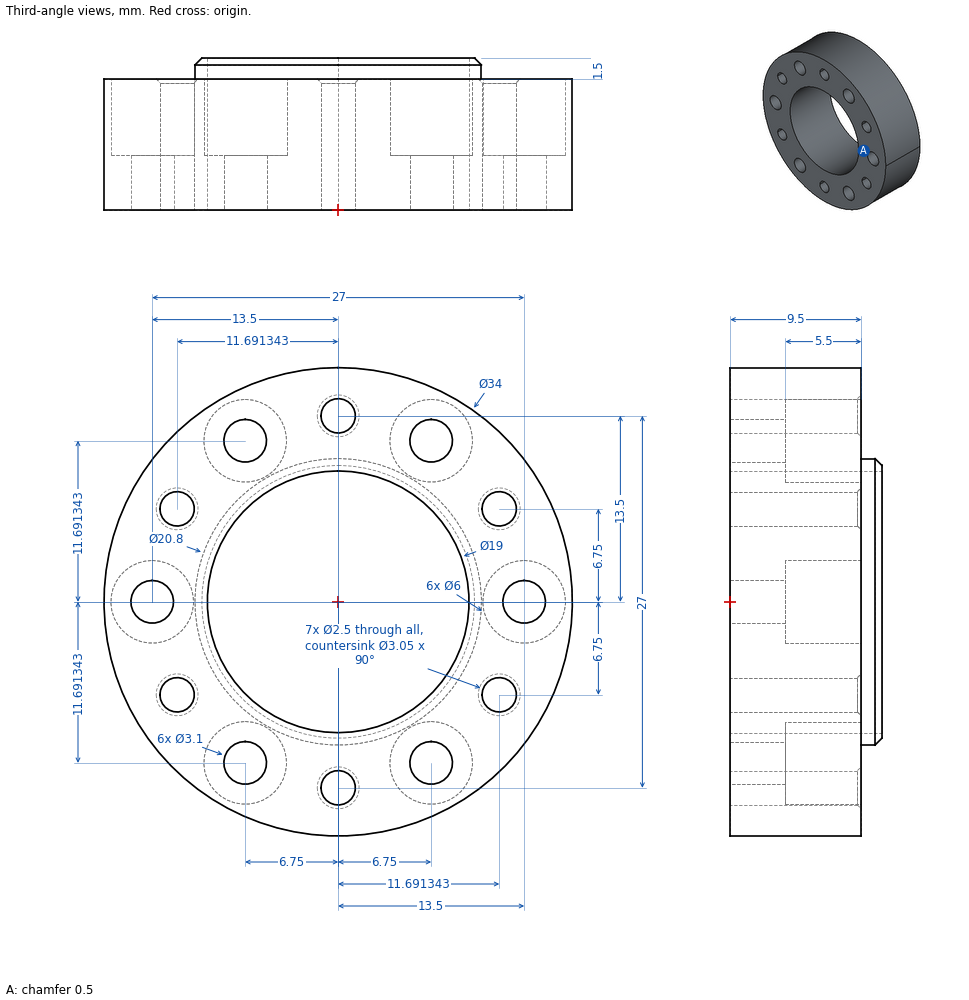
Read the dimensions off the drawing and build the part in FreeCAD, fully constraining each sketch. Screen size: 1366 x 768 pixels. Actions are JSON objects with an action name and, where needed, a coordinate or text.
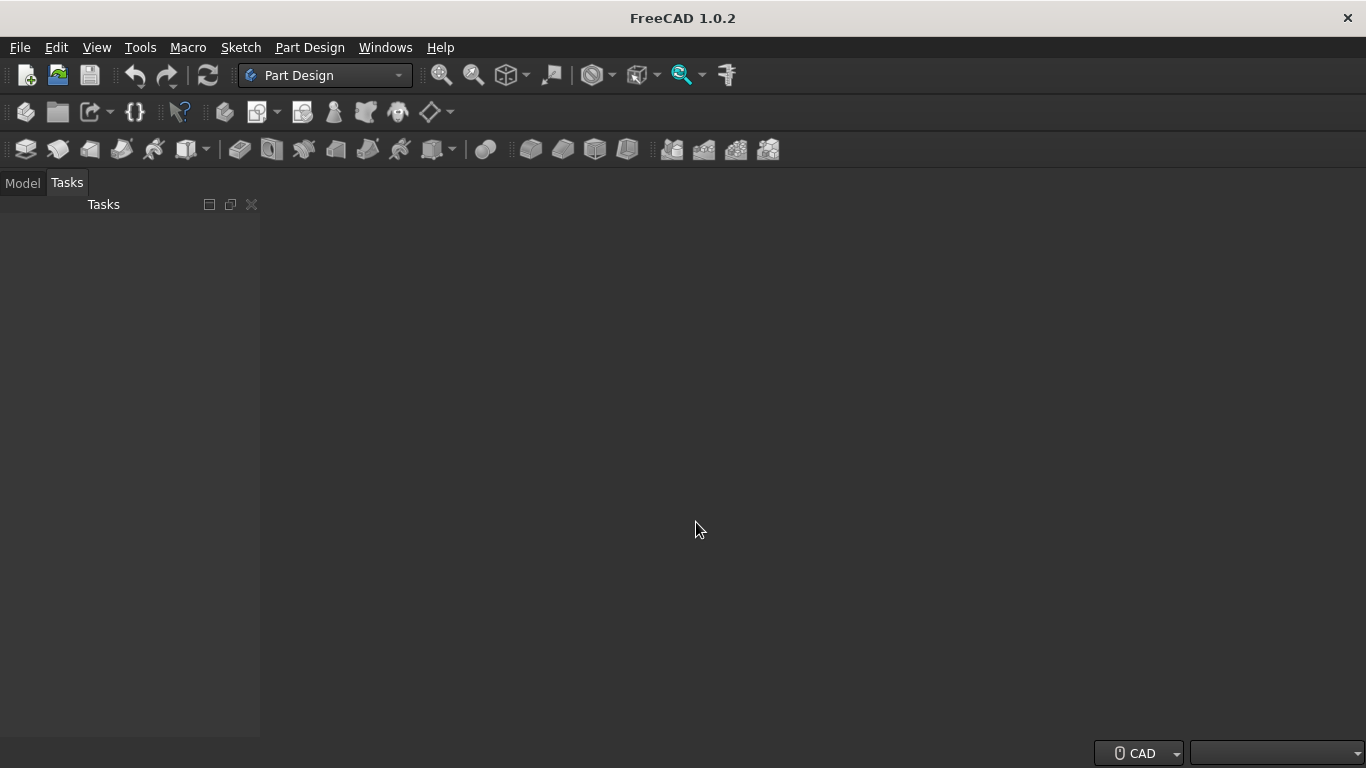
{"action": "left_click", "coordinate": [26, 76]}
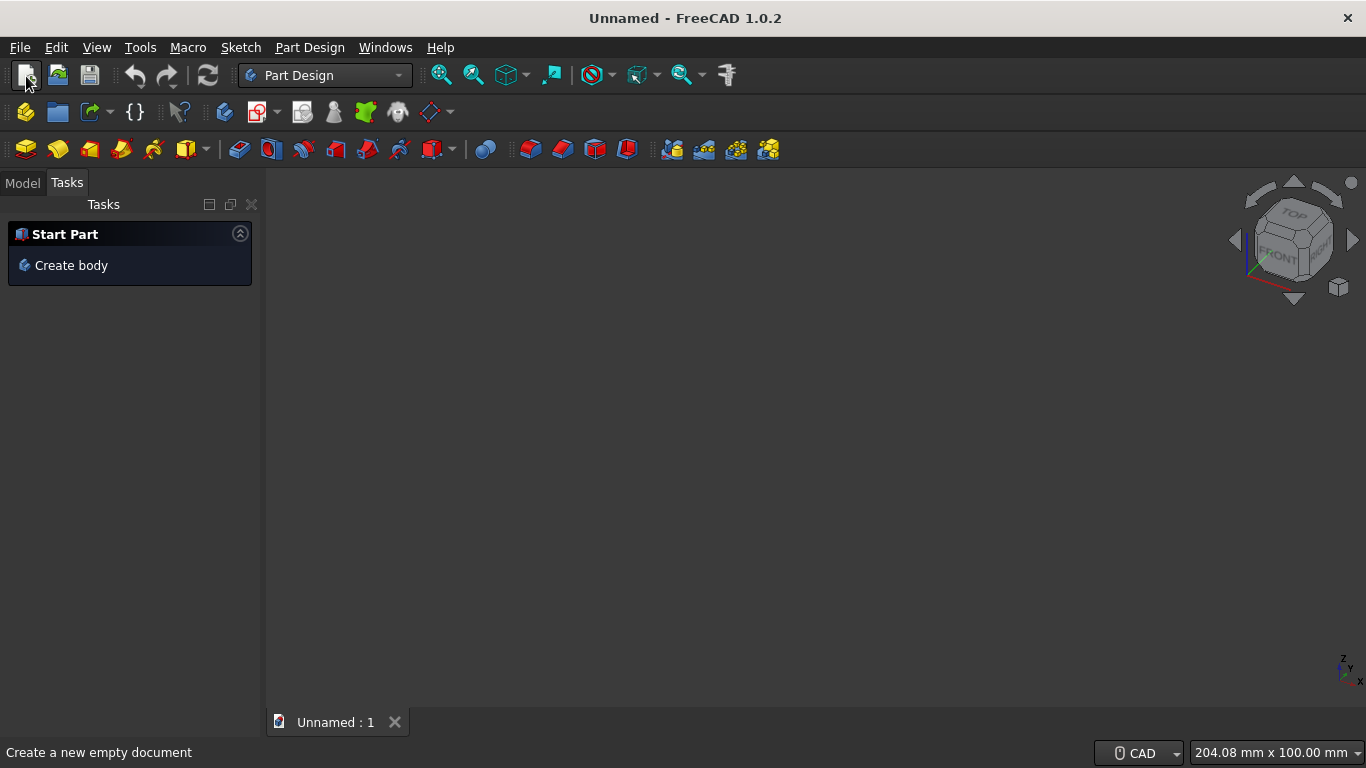
{"action": "left_click", "coordinate": [258, 112]}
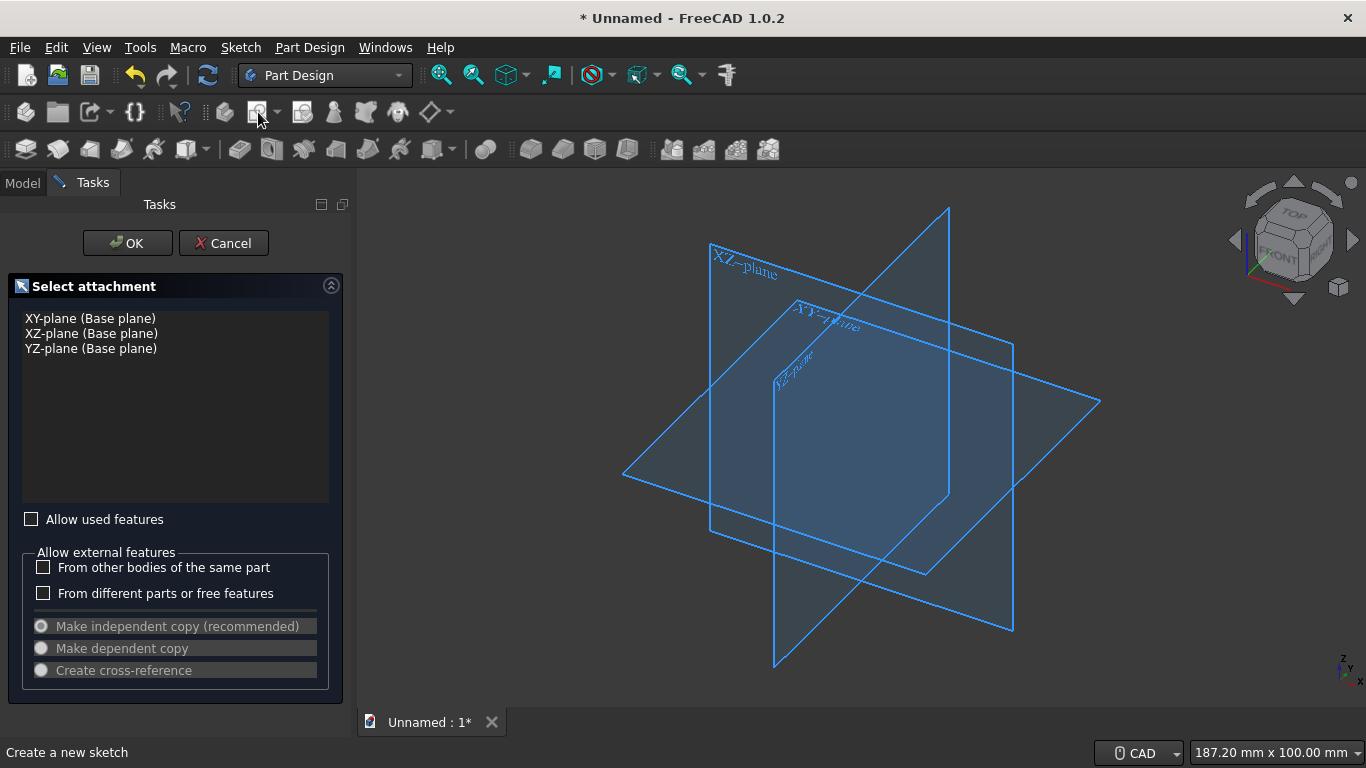
{"action": "left_click", "coordinate": [82, 334]}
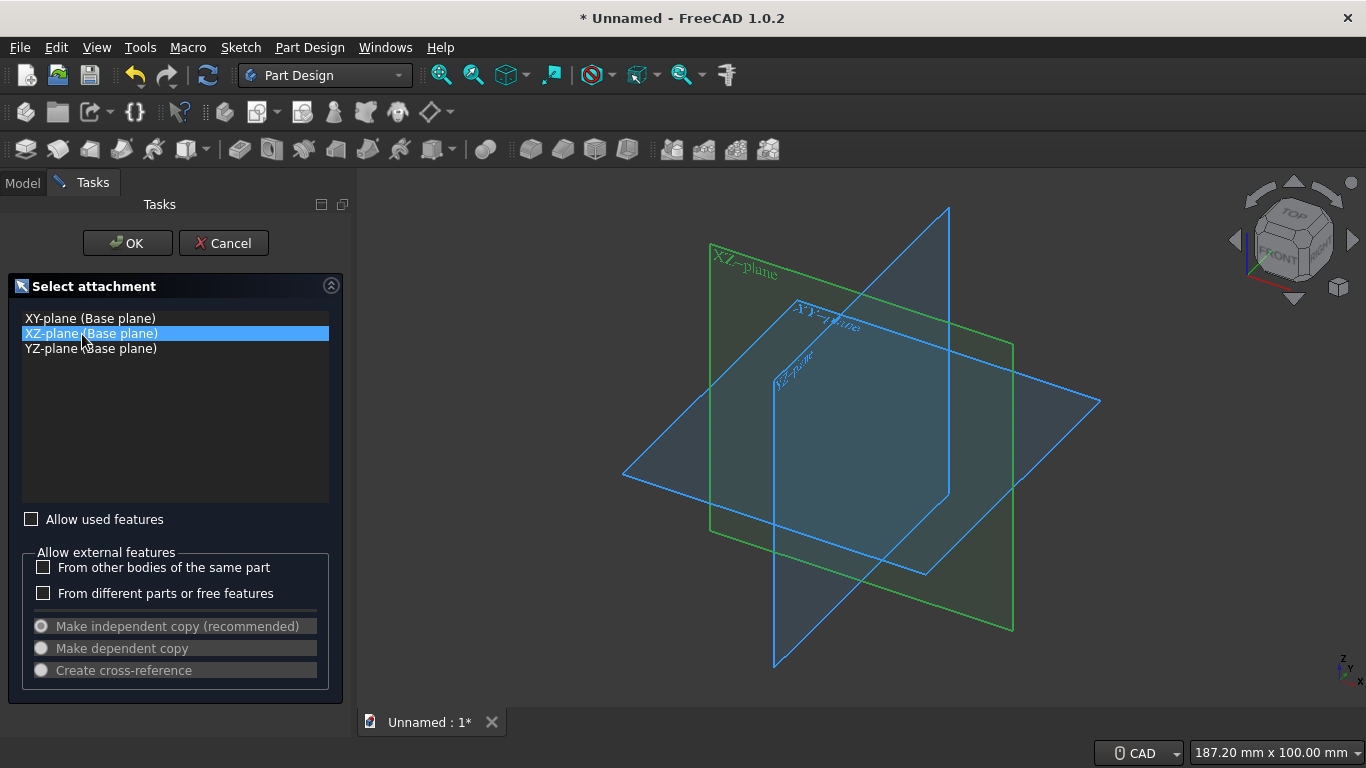
{"action": "left_click", "coordinate": [128, 243]}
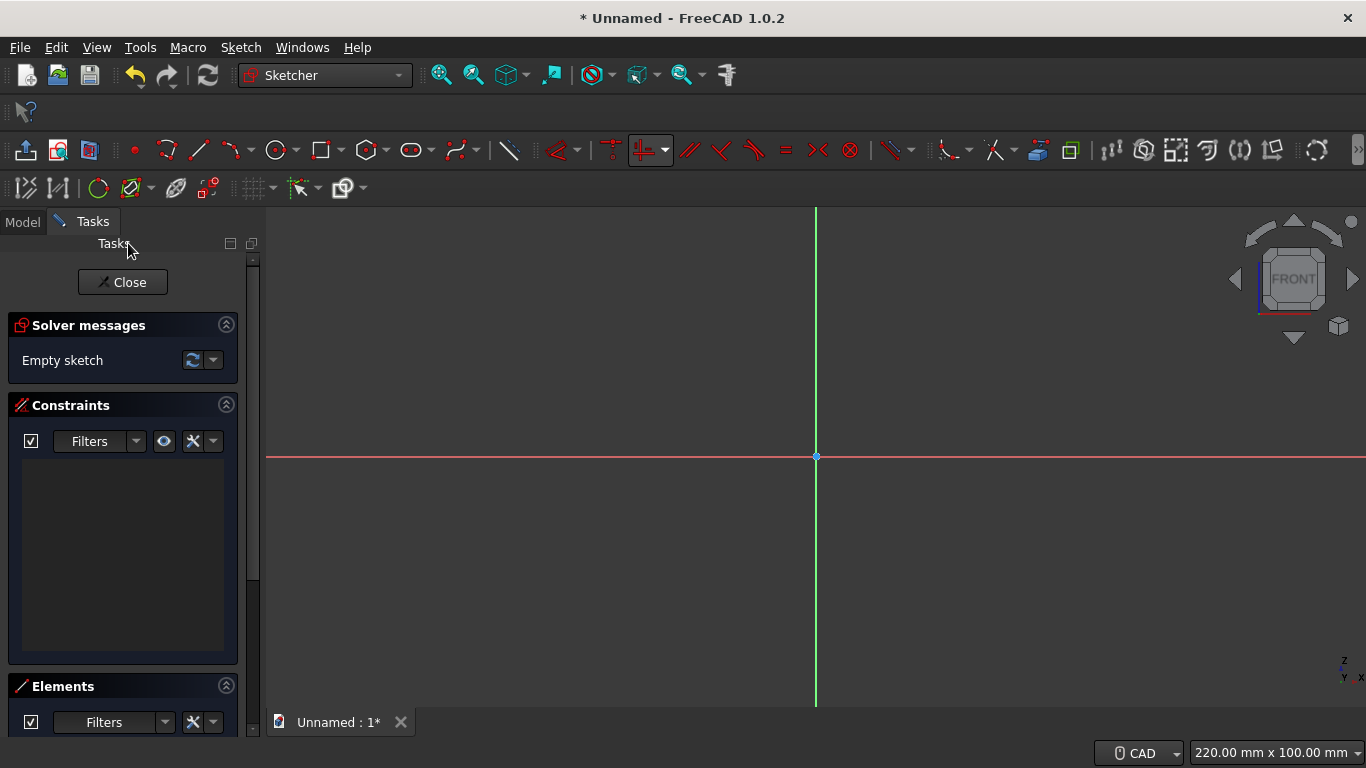
{"action": "scroll", "coordinate": [899, 457], "scroll_direction": "up", "scroll_amount": 3}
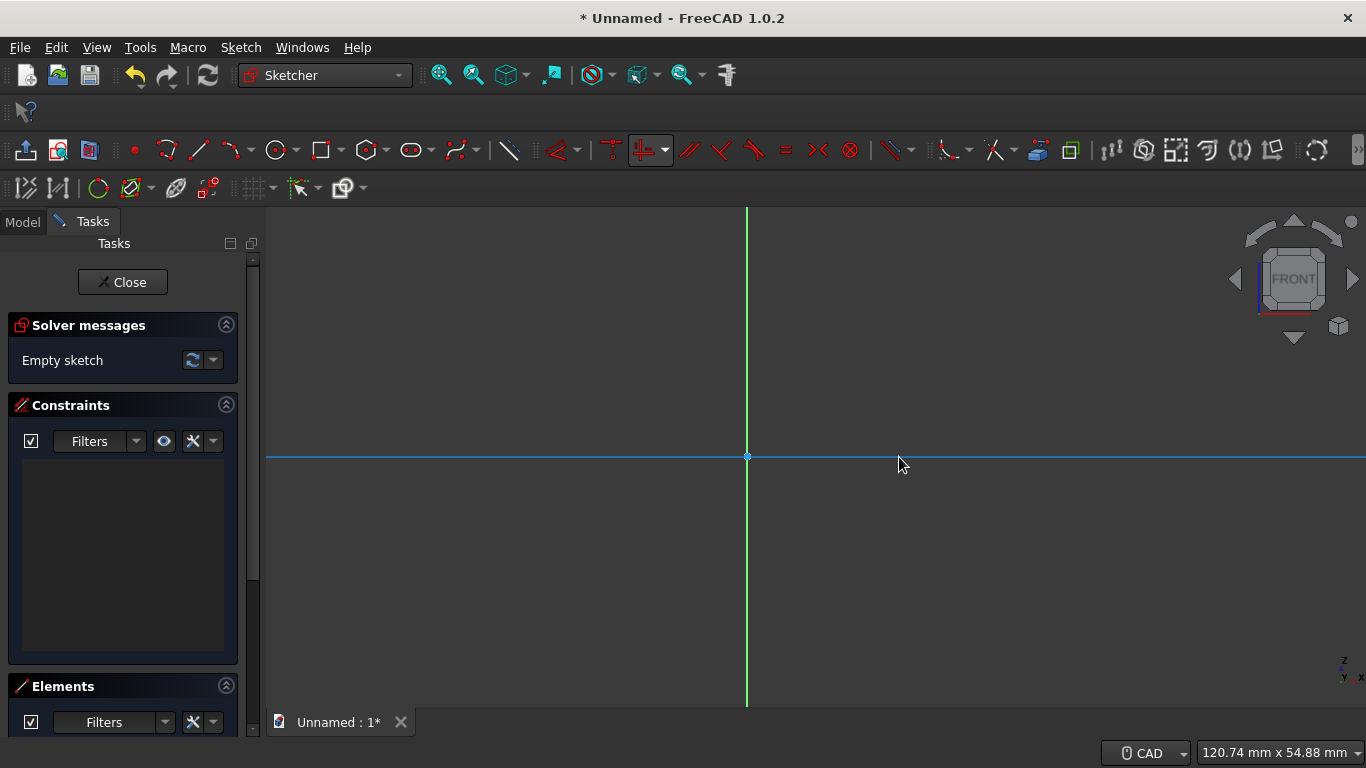
{"action": "left_click", "coordinate": [276, 150]}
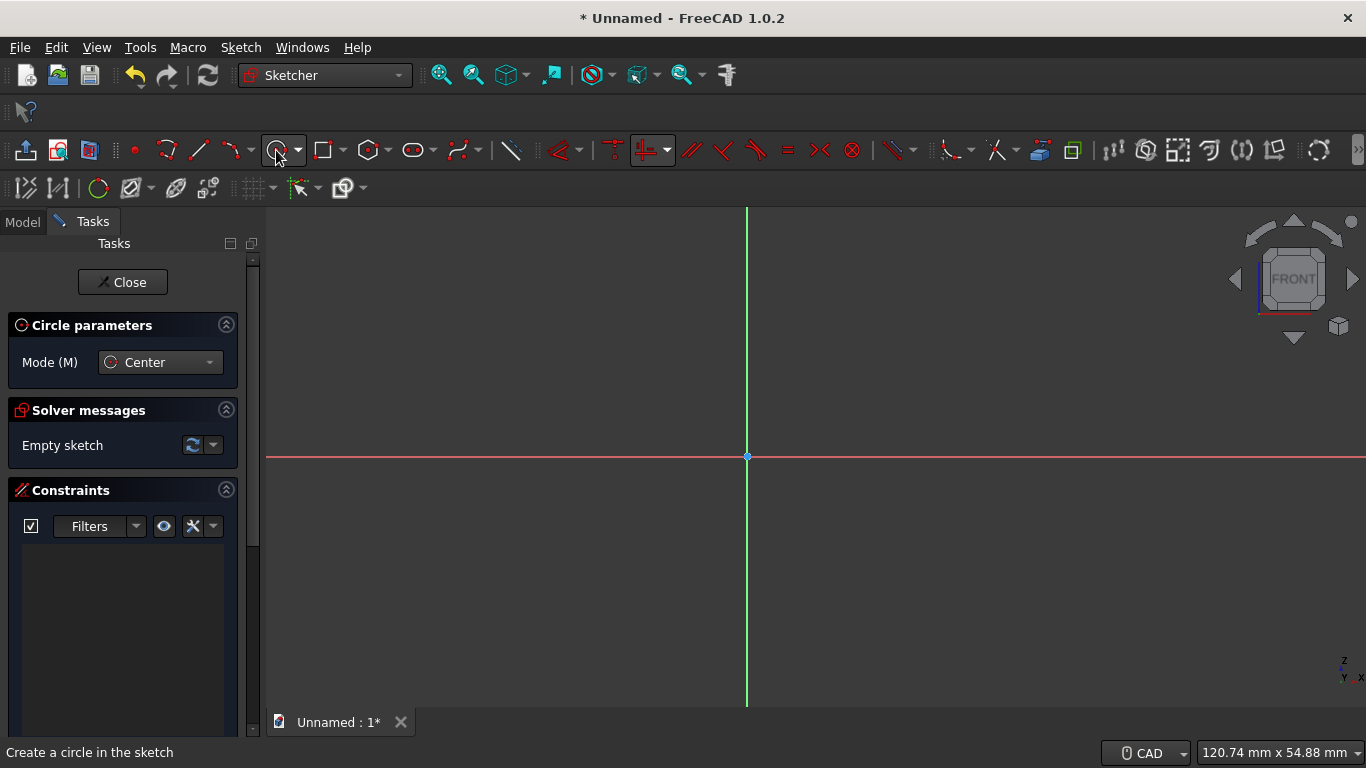
{"action": "left_click", "coordinate": [747, 457]}
{"action": "mouse_move", "coordinate": [857, 347]}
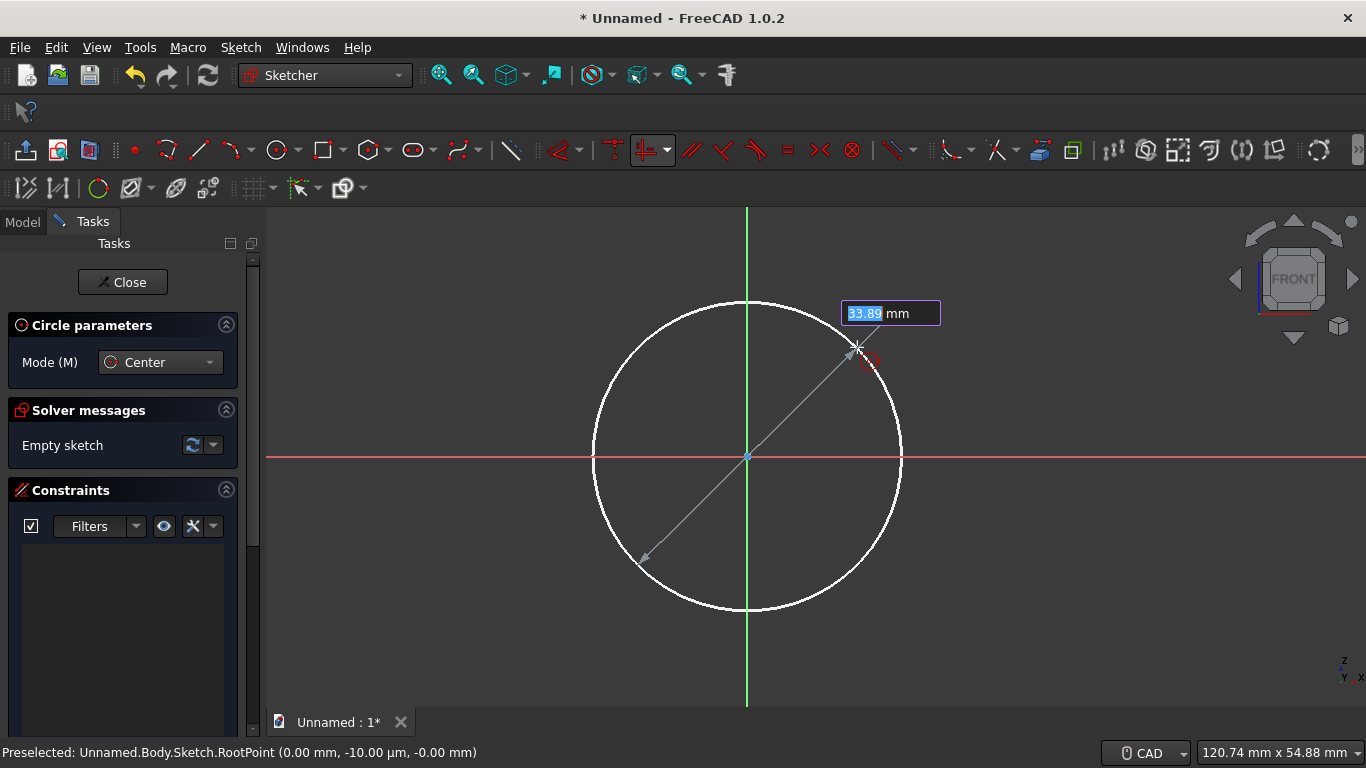
{"action": "type", "text": "34"}
{"action": "key", "text": "Return"}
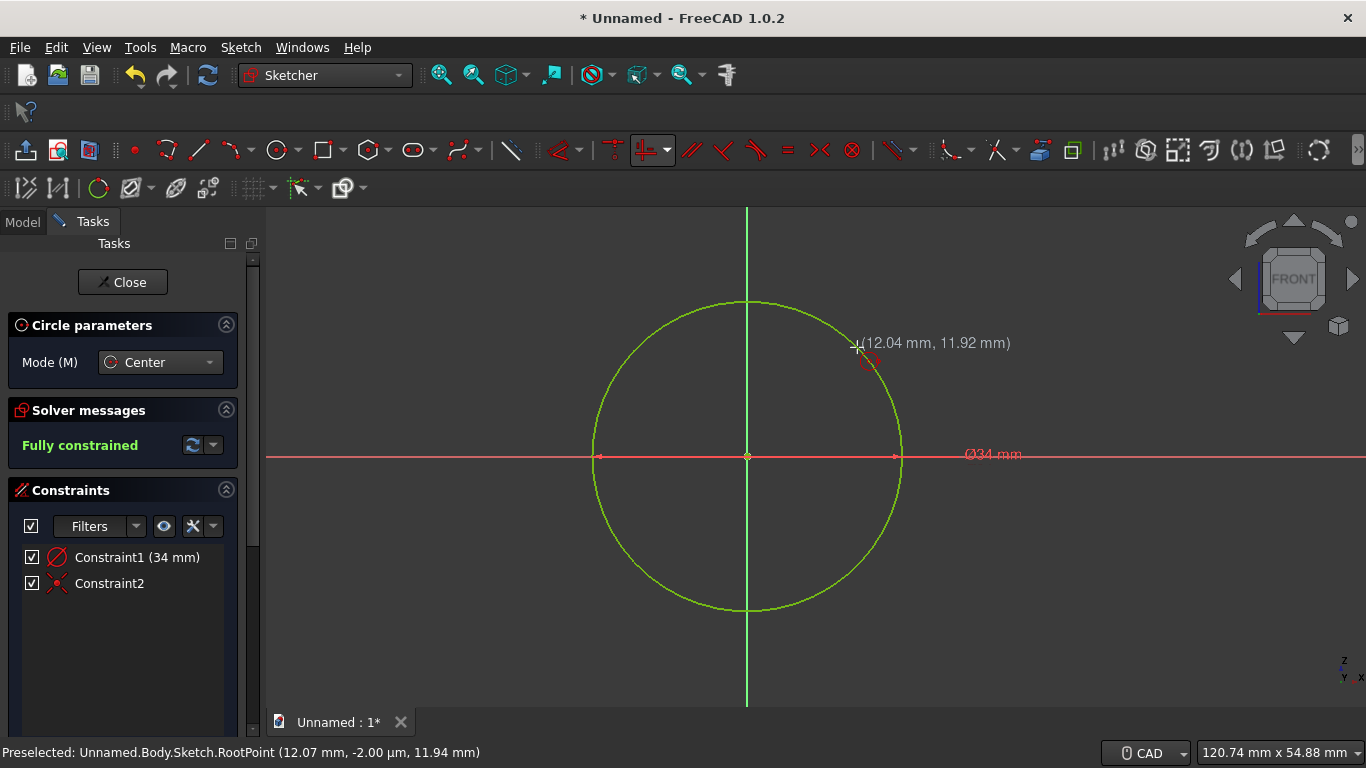
{"action": "scroll", "coordinate": [686, 563], "scroll_direction": "up", "scroll_amount": 3}